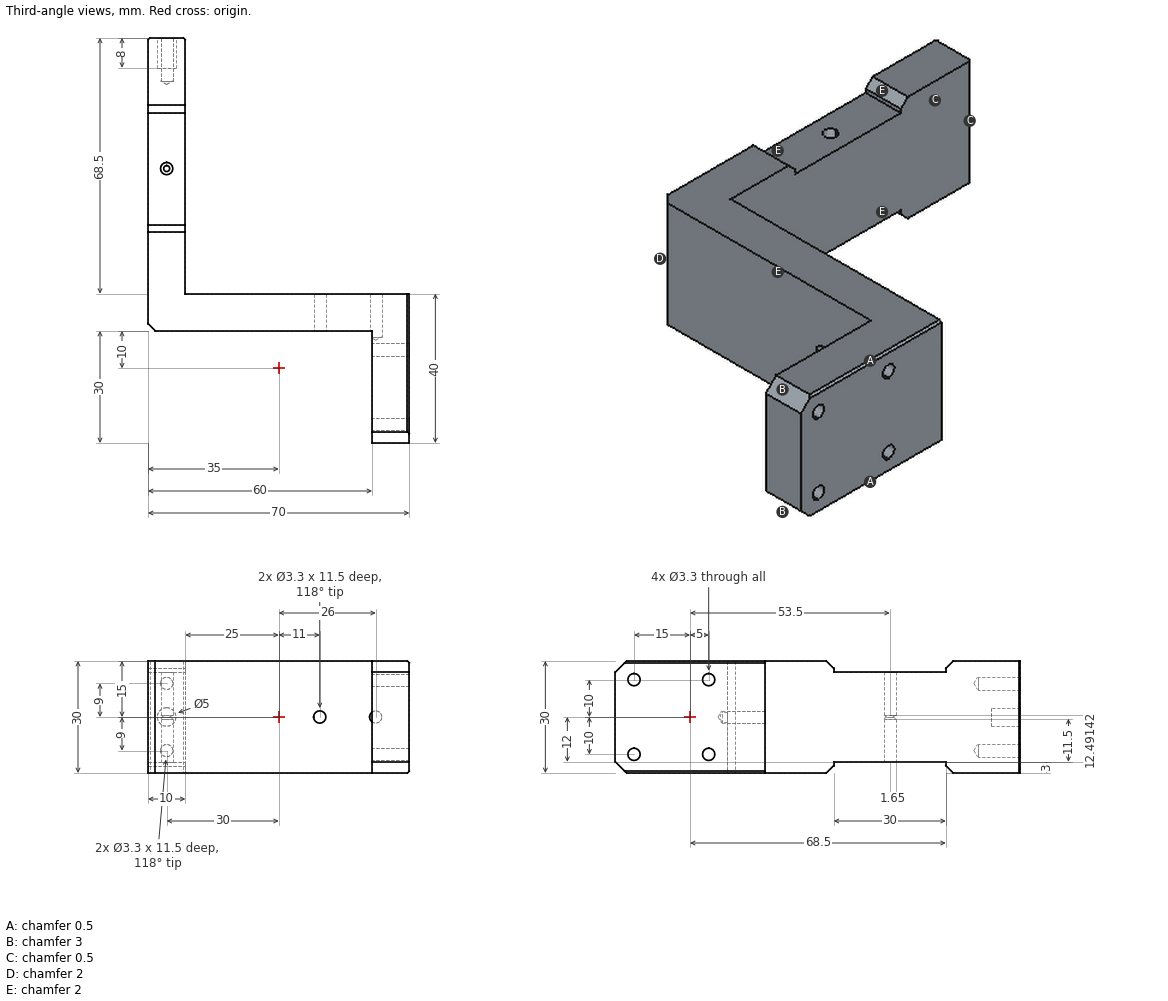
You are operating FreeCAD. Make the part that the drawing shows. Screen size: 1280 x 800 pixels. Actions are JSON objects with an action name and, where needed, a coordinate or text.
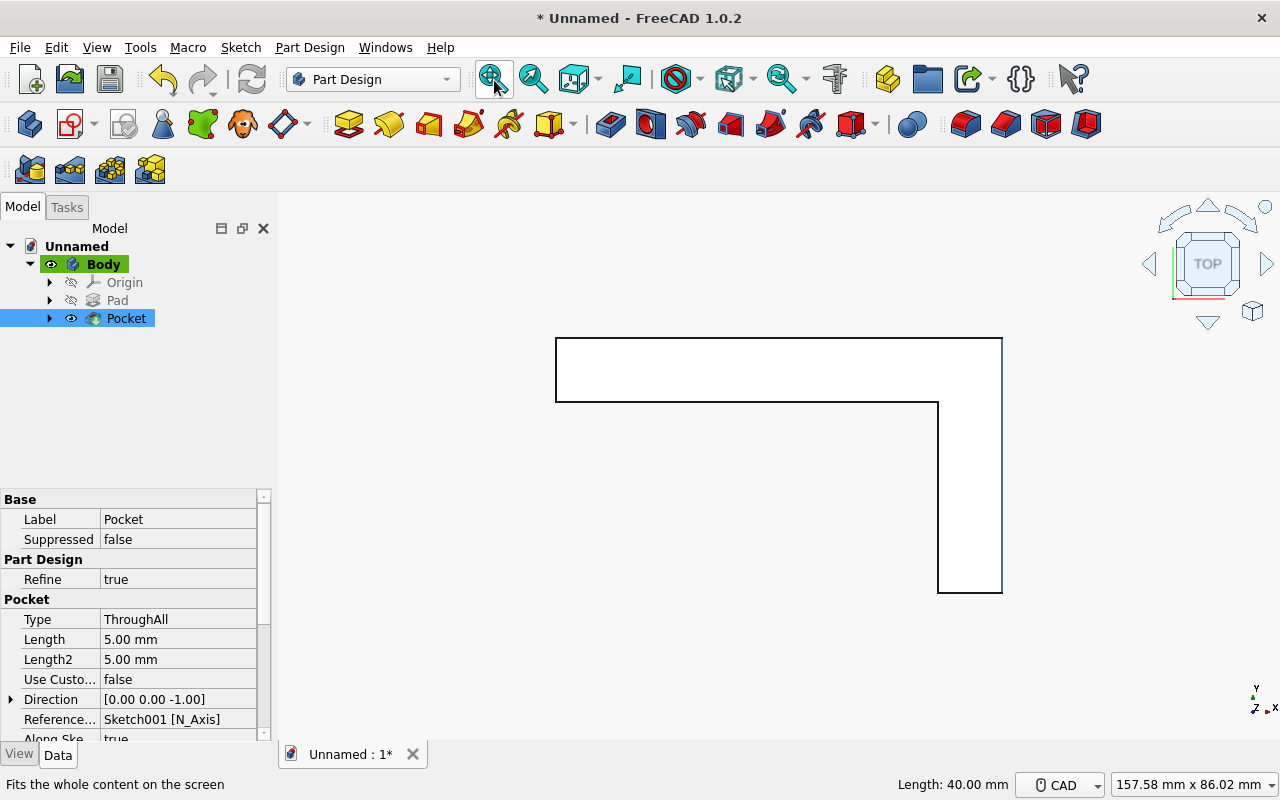
{"action": "key", "text": "1"}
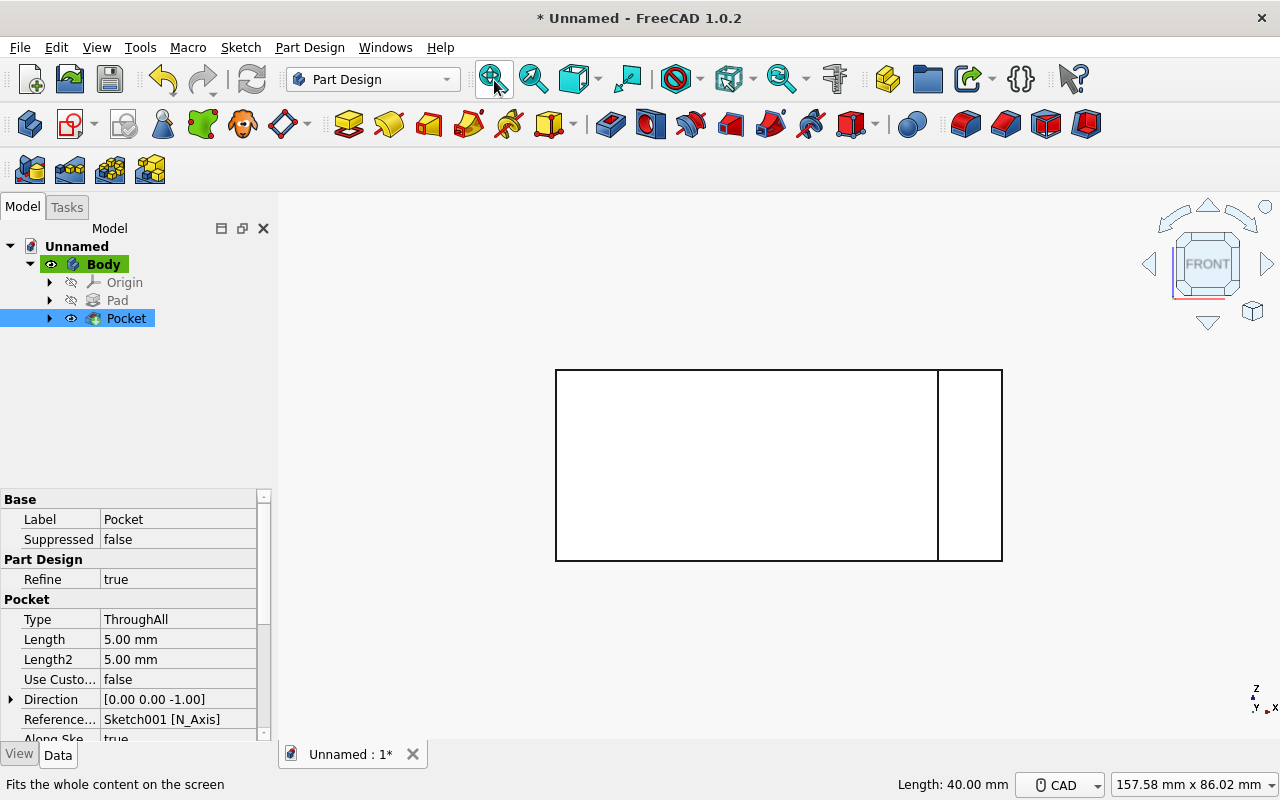
{"action": "key", "text": "v f"}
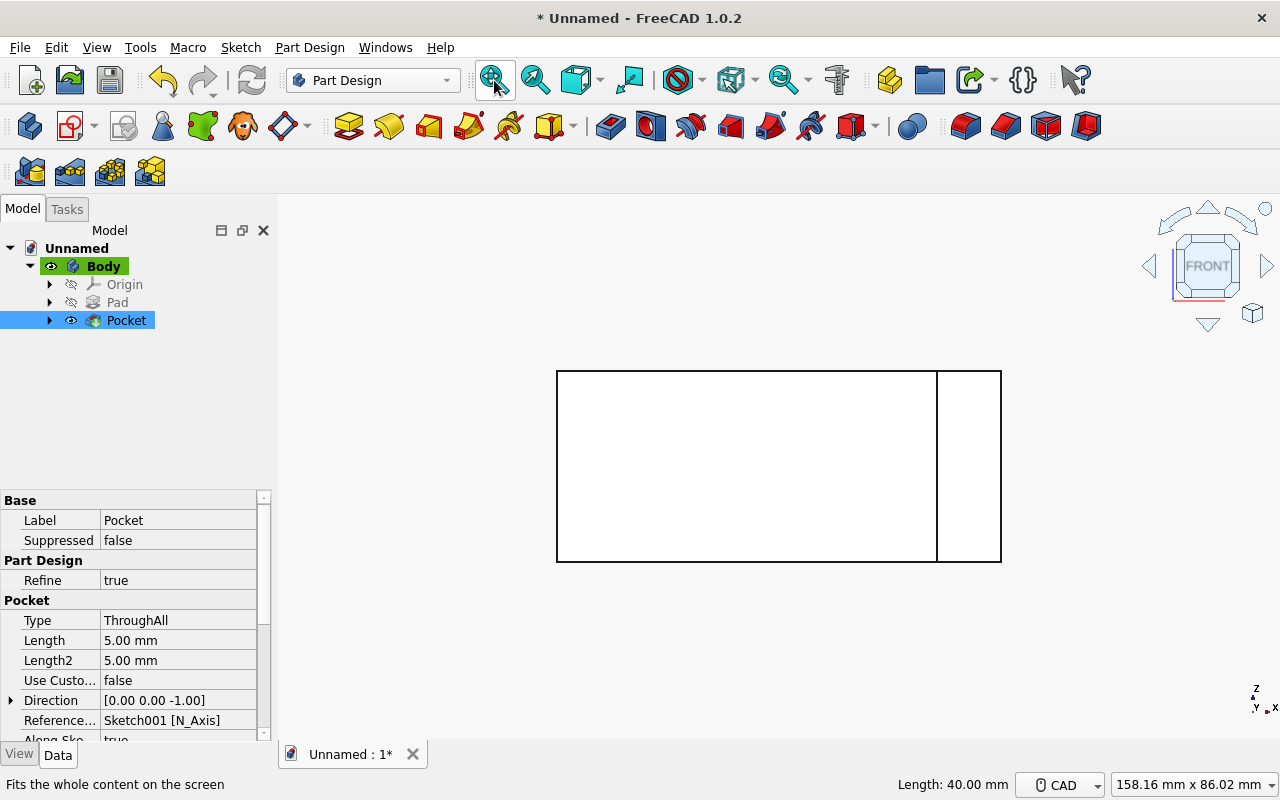
{"action": "key", "text": "3"}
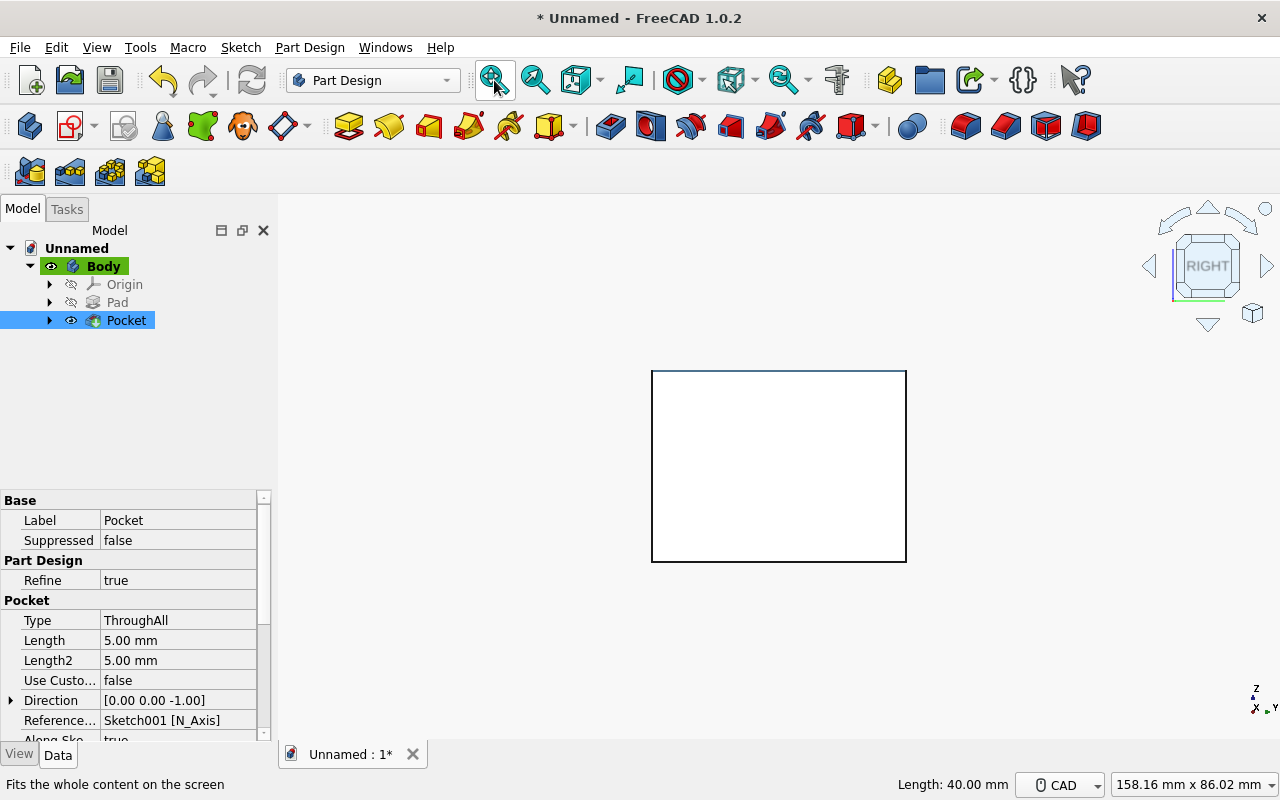
{"action": "left_click", "coordinate": [496, 80]}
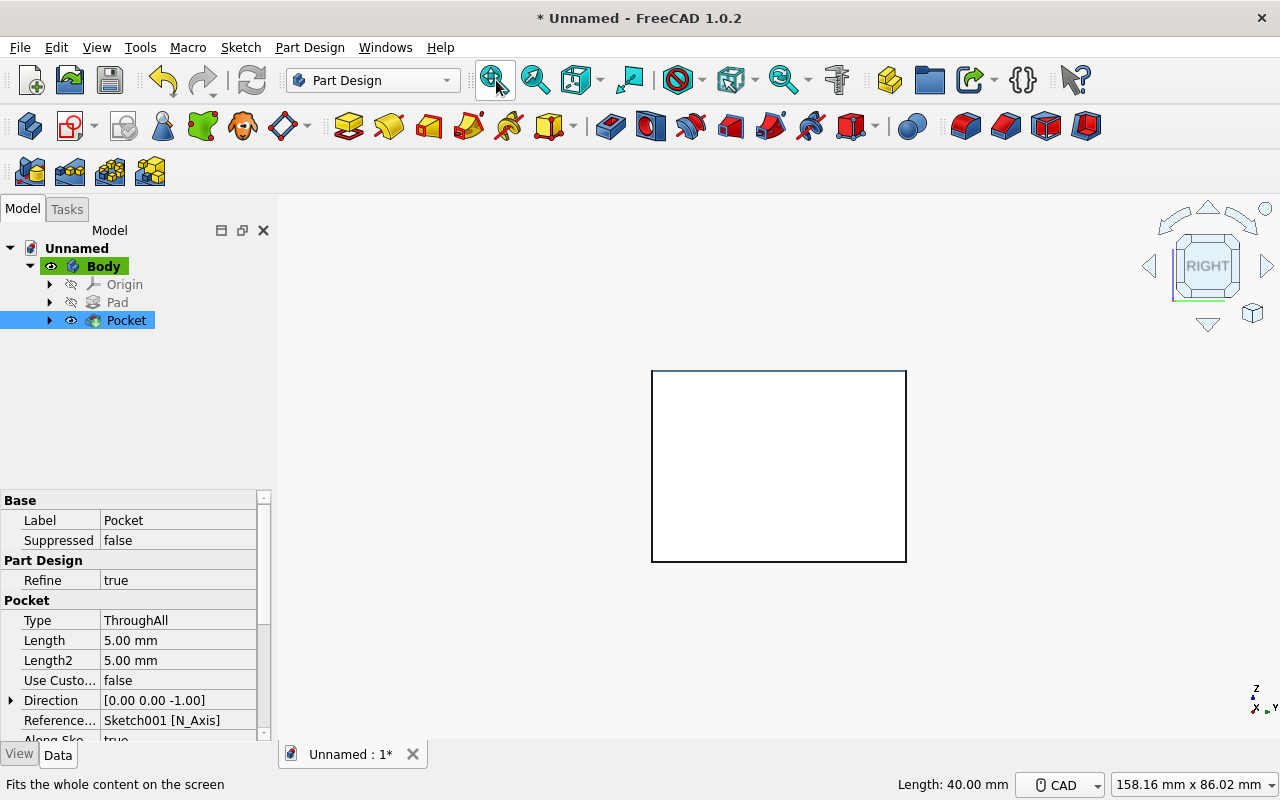
{"action": "left_click", "coordinate": [779, 561], "text": "ctrl"}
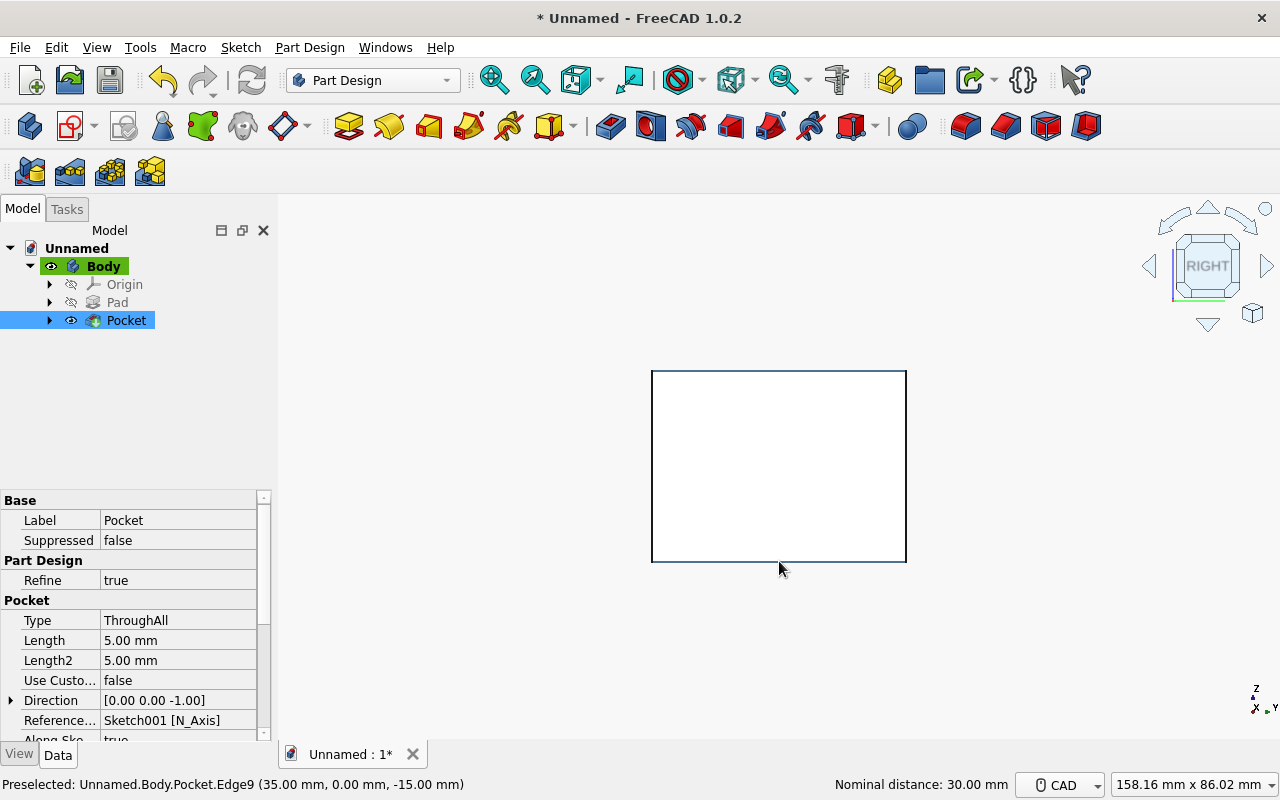
{"action": "left_click", "coordinate": [1006, 126]}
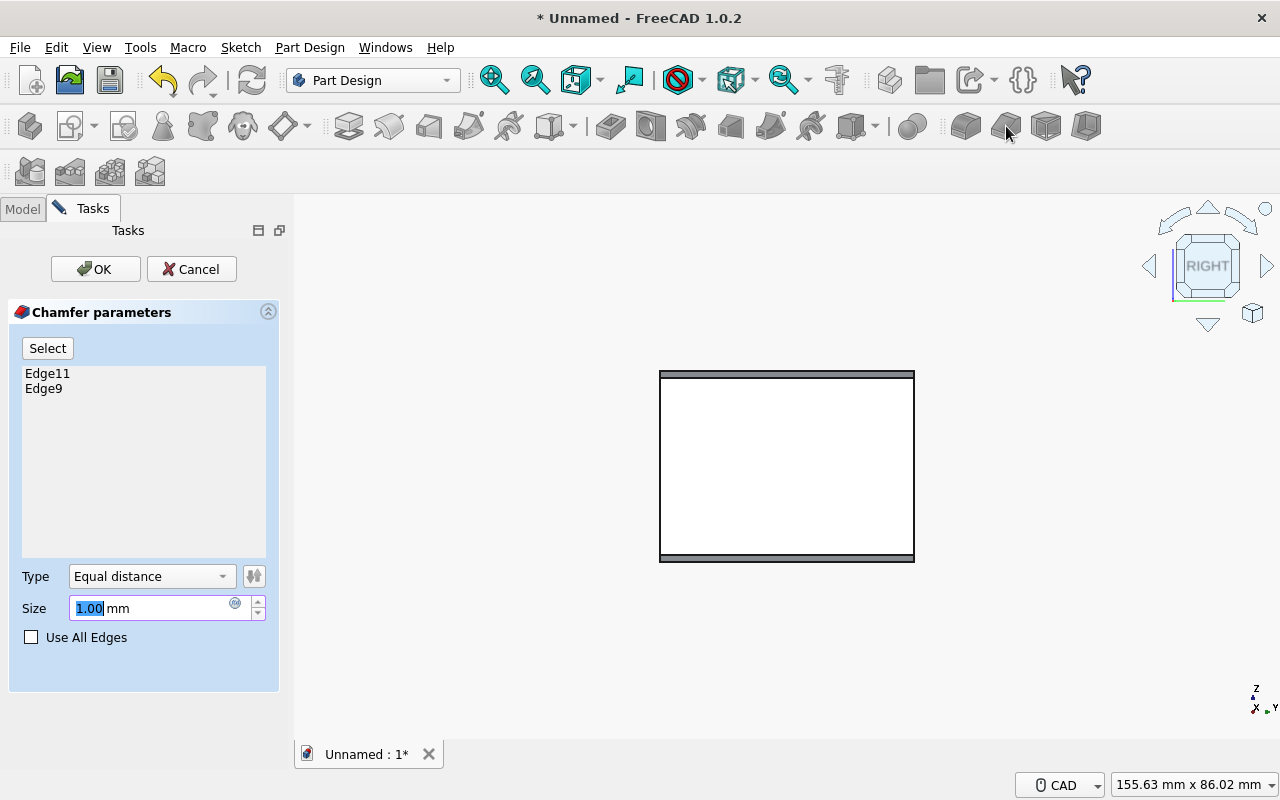
{"action": "type", "text": "0.5"}
{"action": "key", "text": "Tab"}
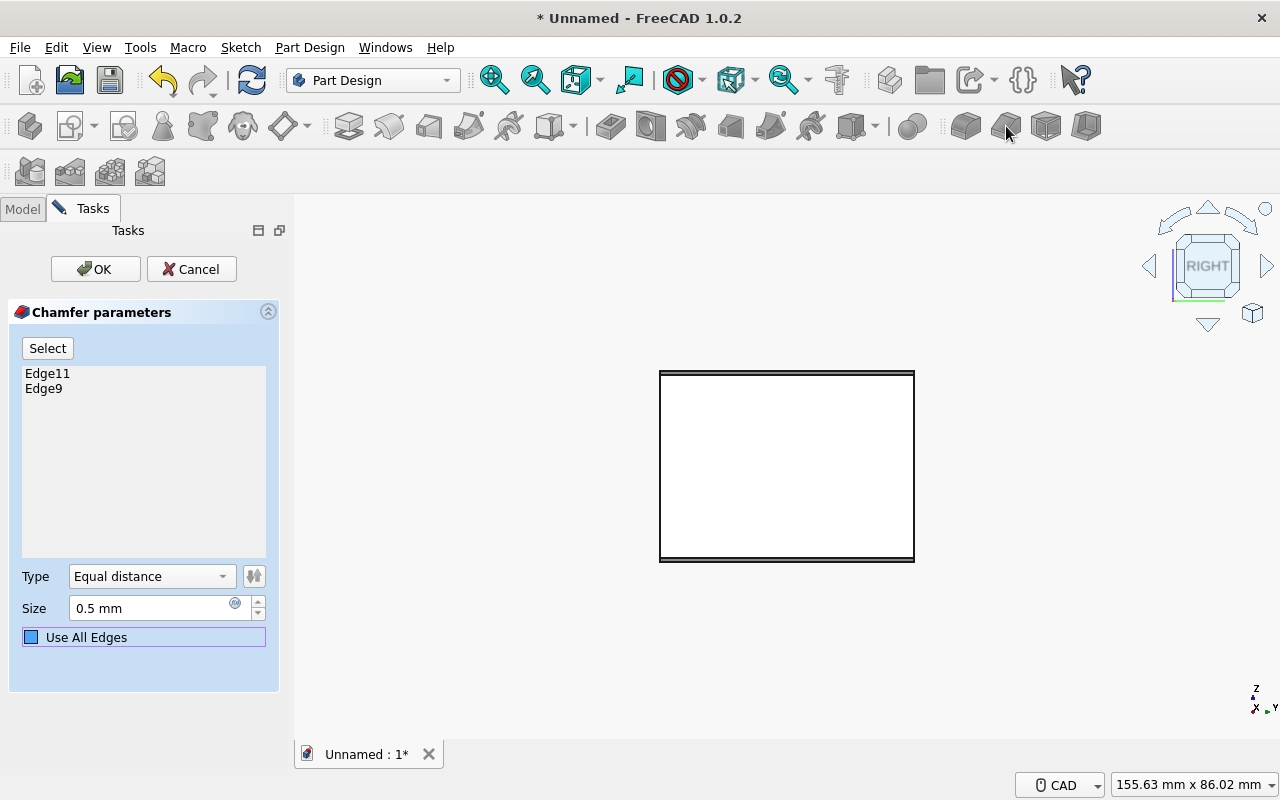
{"action": "left_click", "coordinate": [96, 269]}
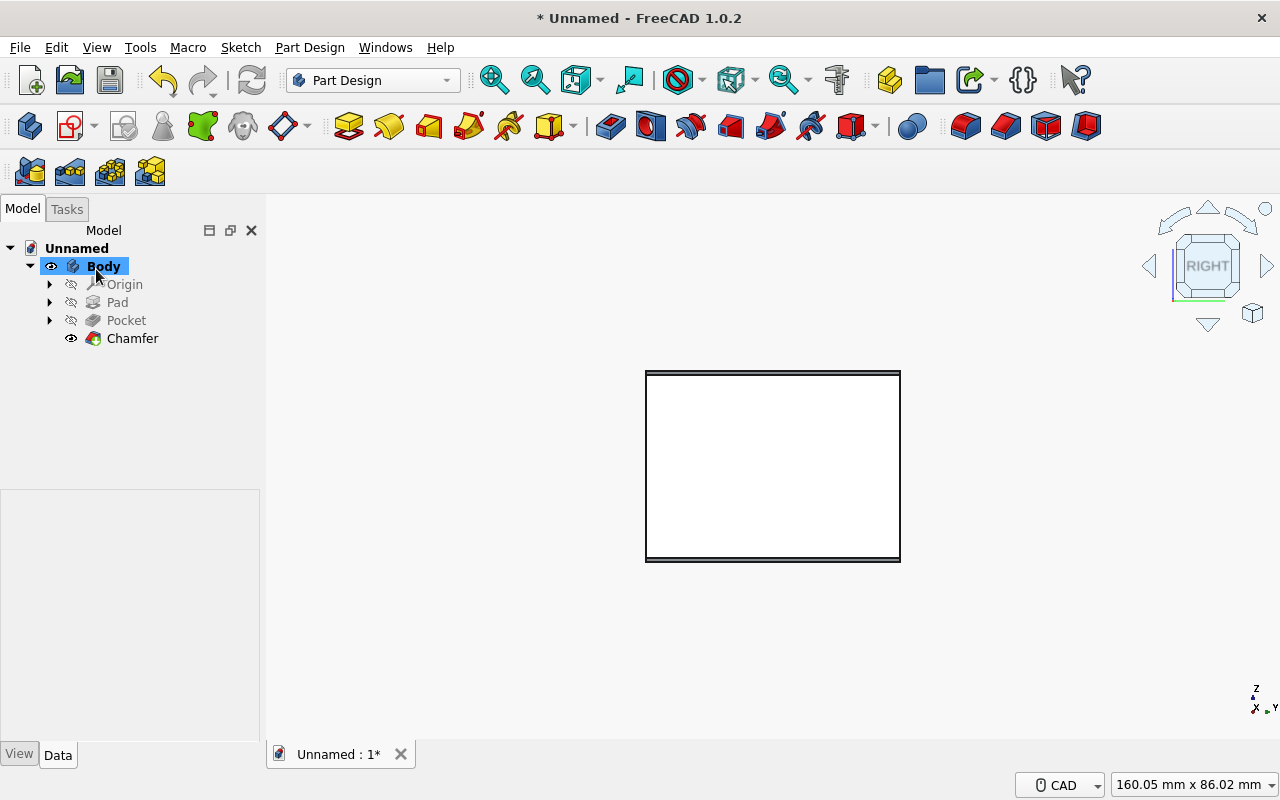
{"action": "left_click", "coordinate": [496, 80]}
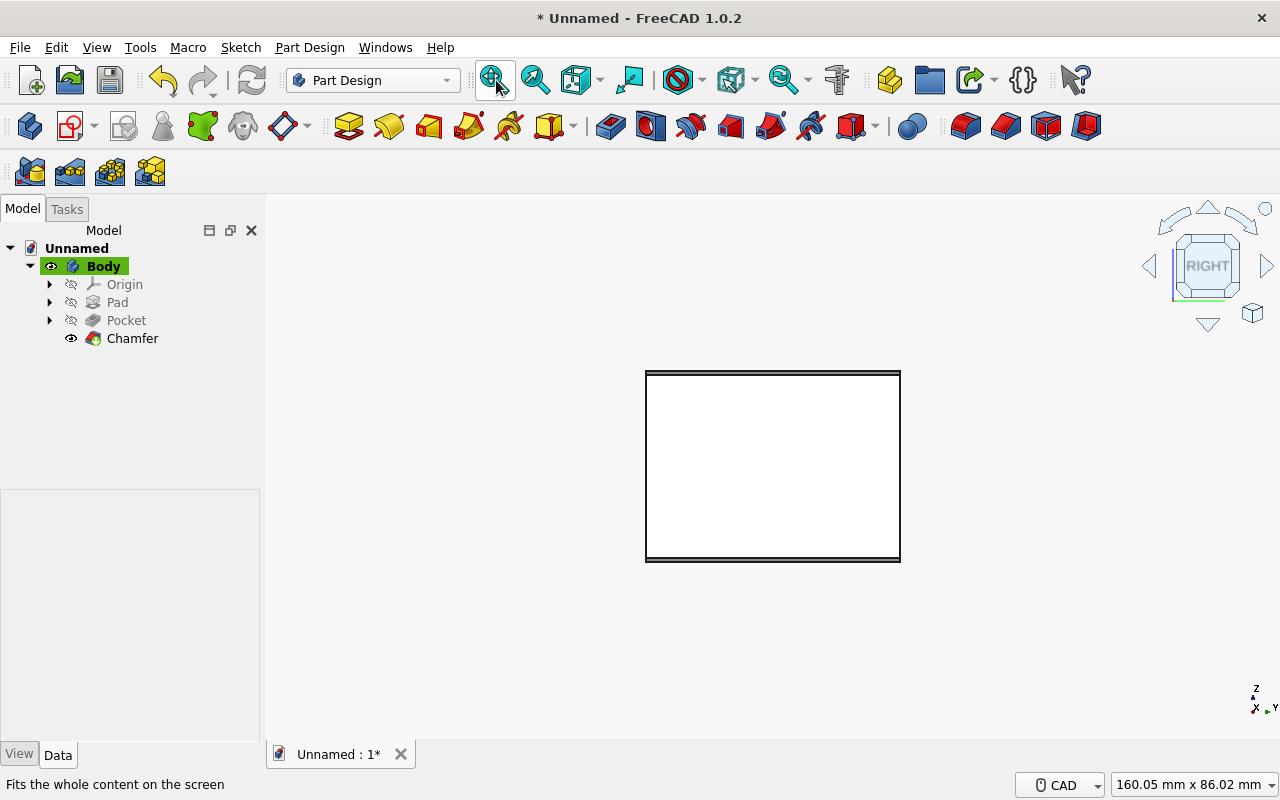
{"action": "key", "text": "4"}